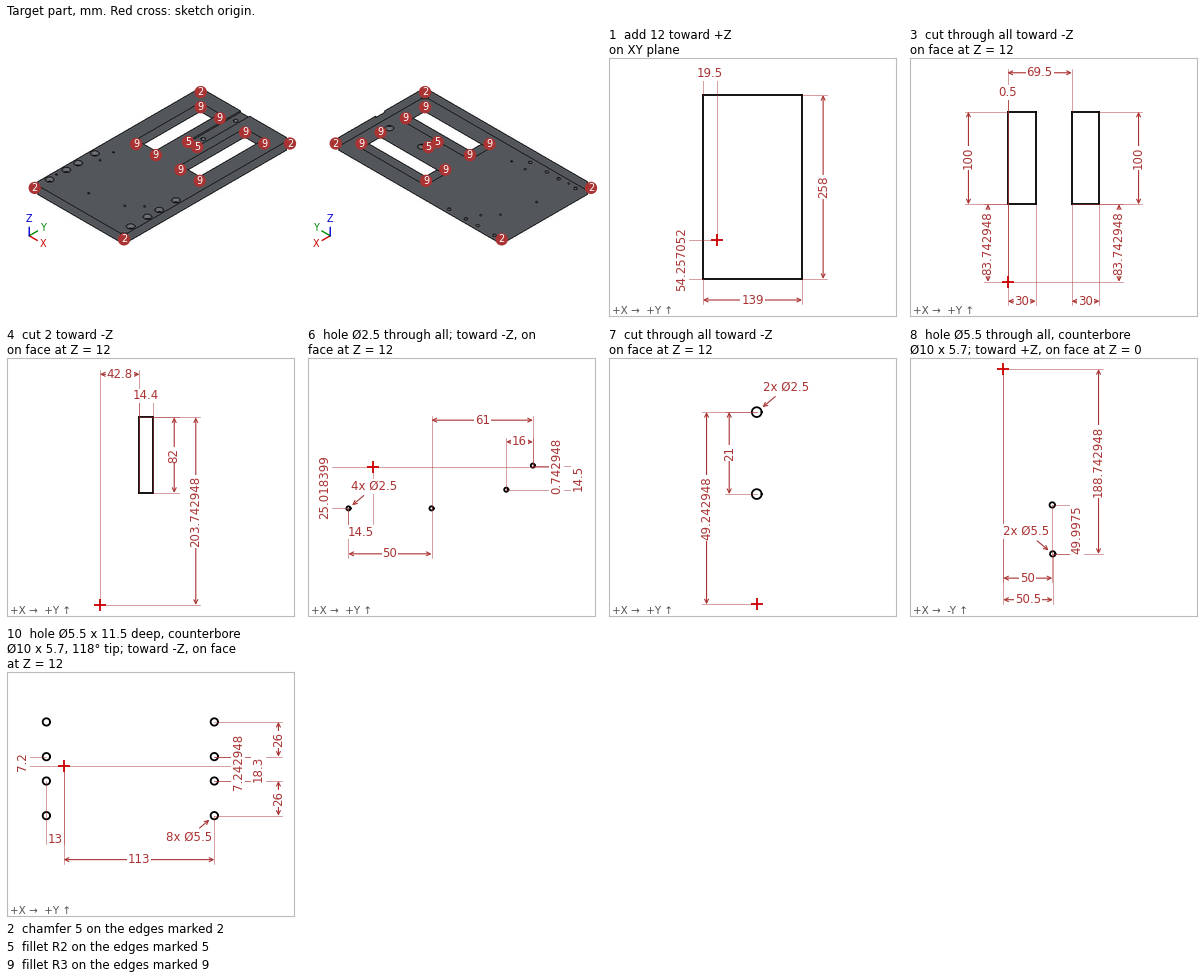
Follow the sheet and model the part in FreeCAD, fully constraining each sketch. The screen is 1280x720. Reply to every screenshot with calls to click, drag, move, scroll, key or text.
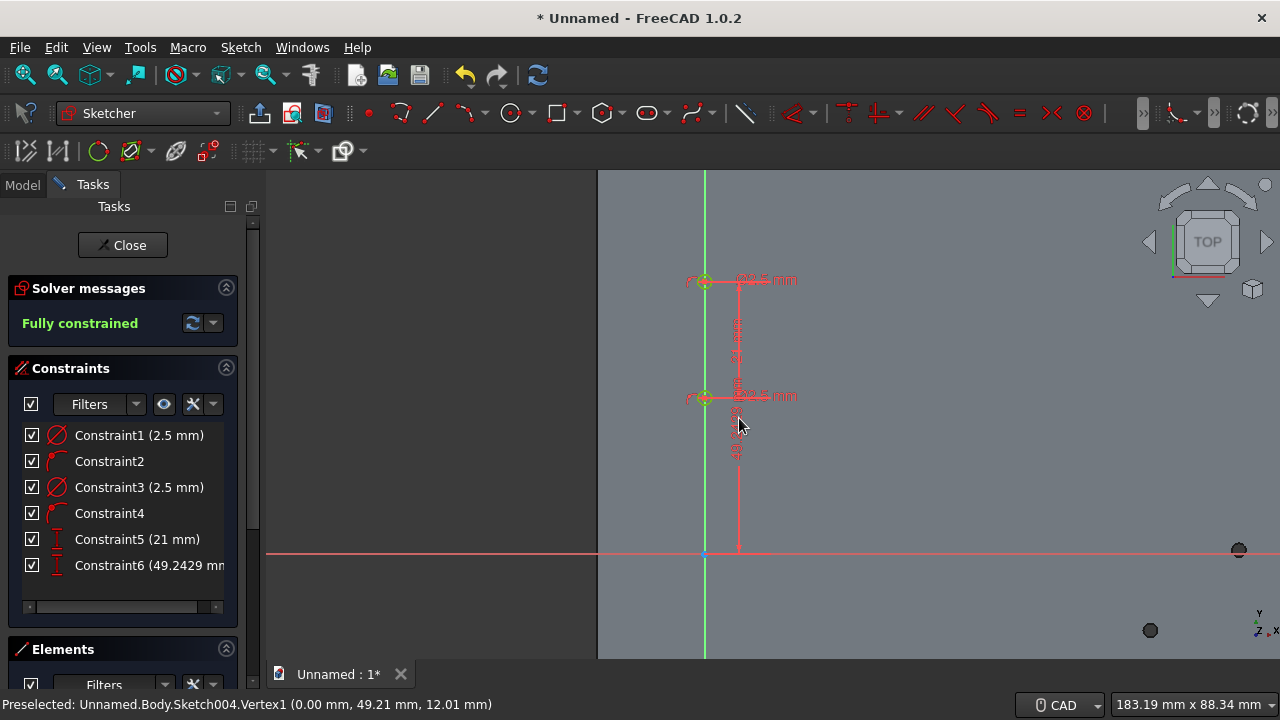
click(123, 245)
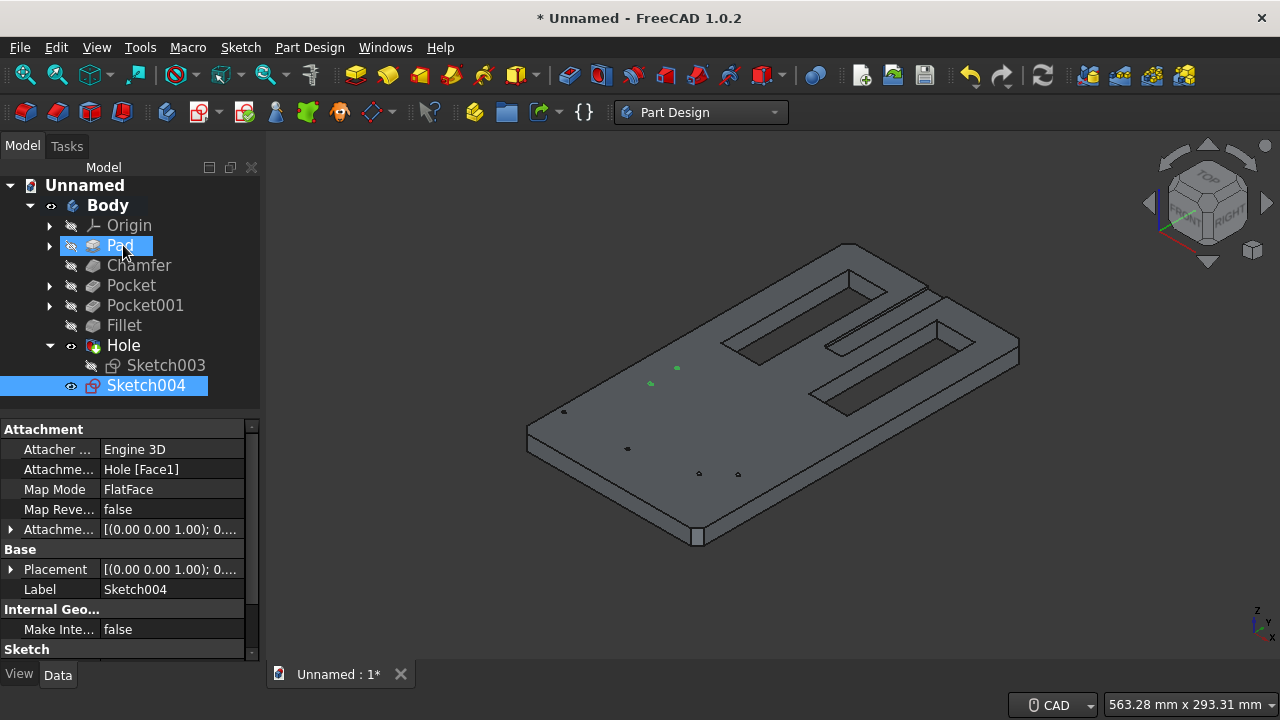
click(570, 76)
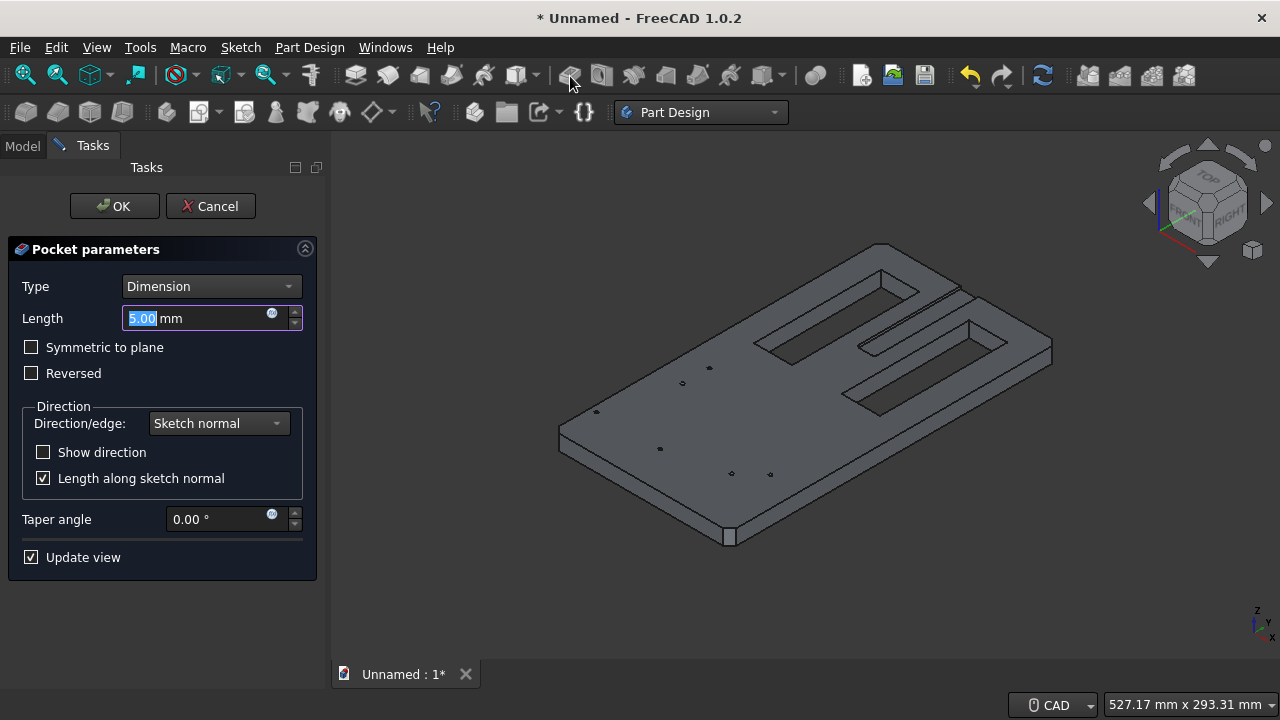
click(212, 286)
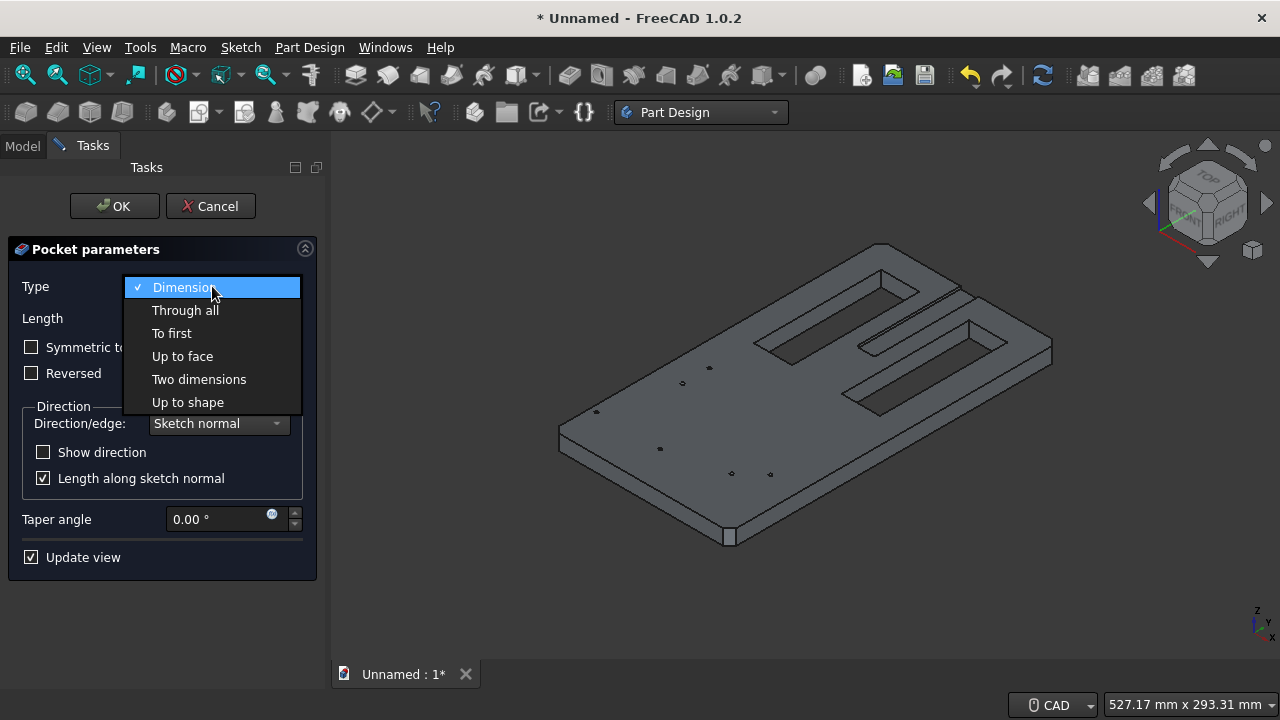
click(212, 310)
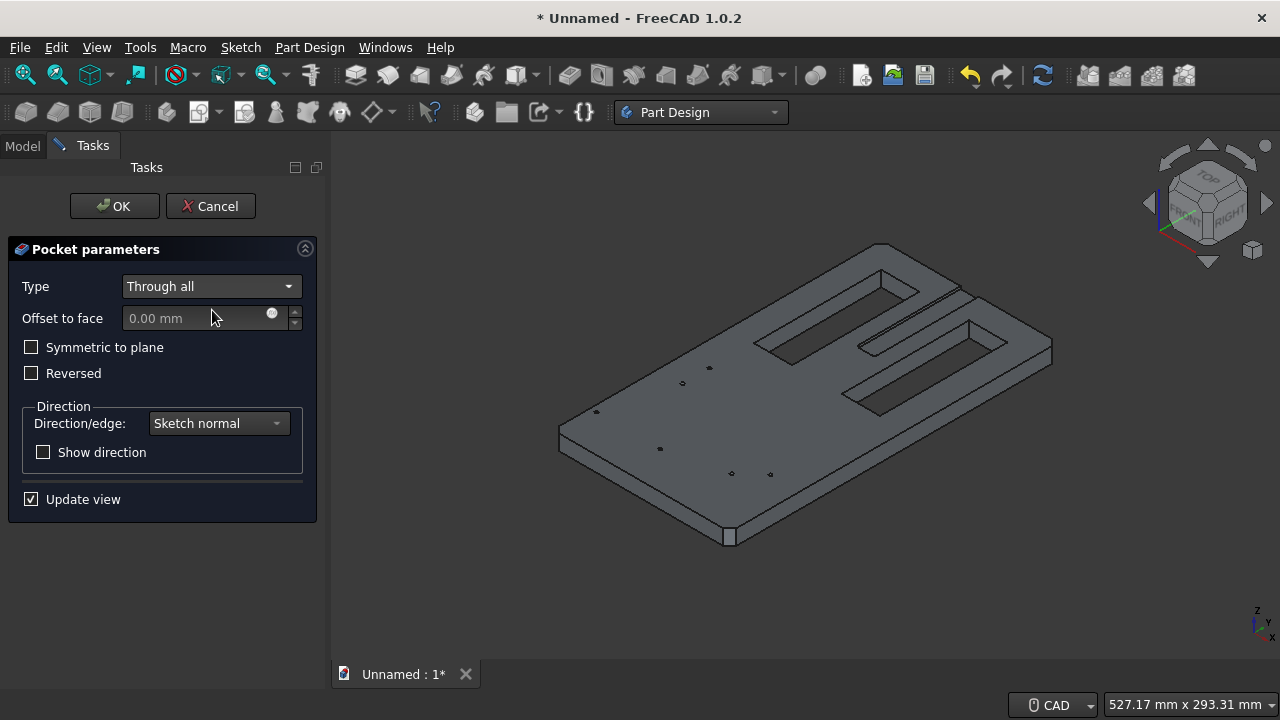
click(115, 206)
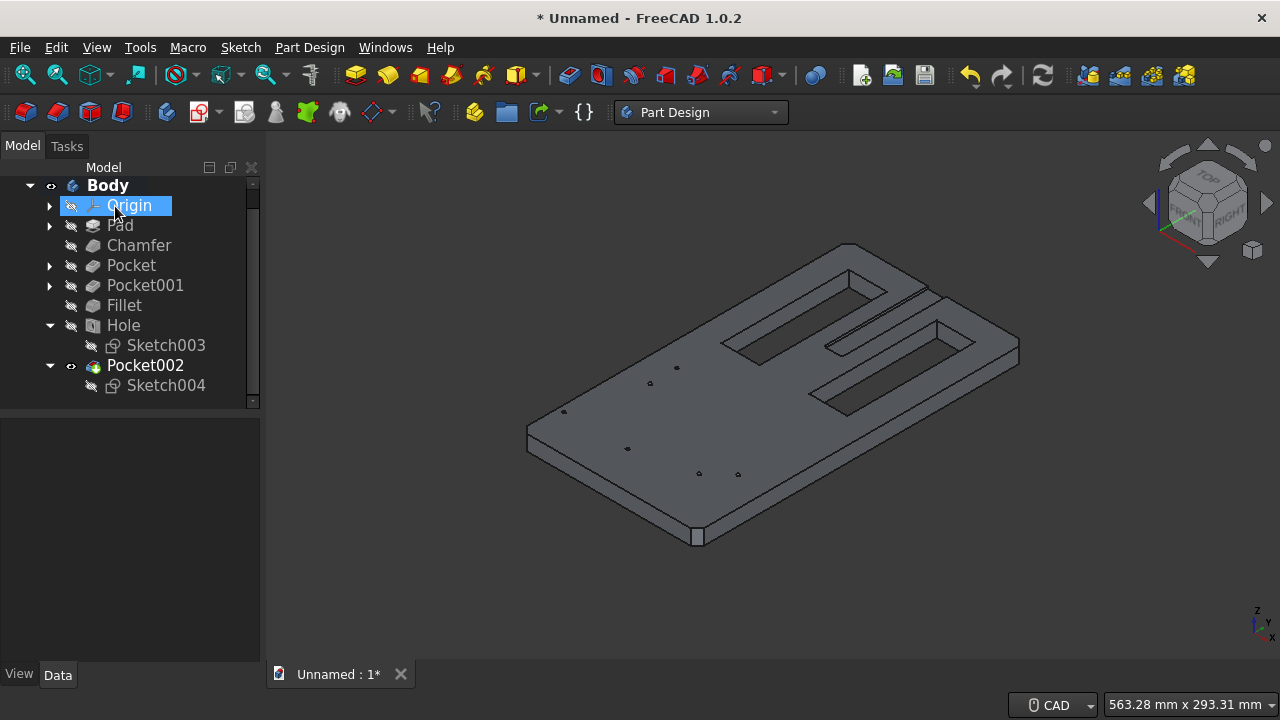
key(5)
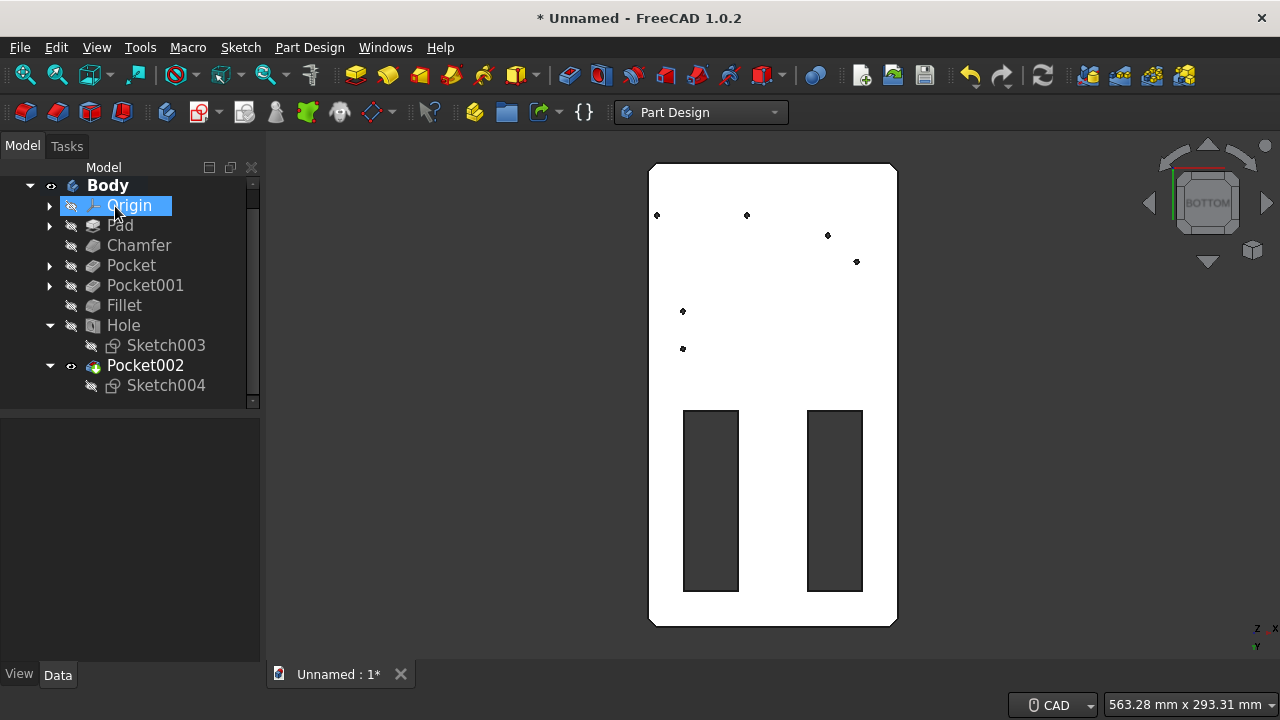
click(773, 328)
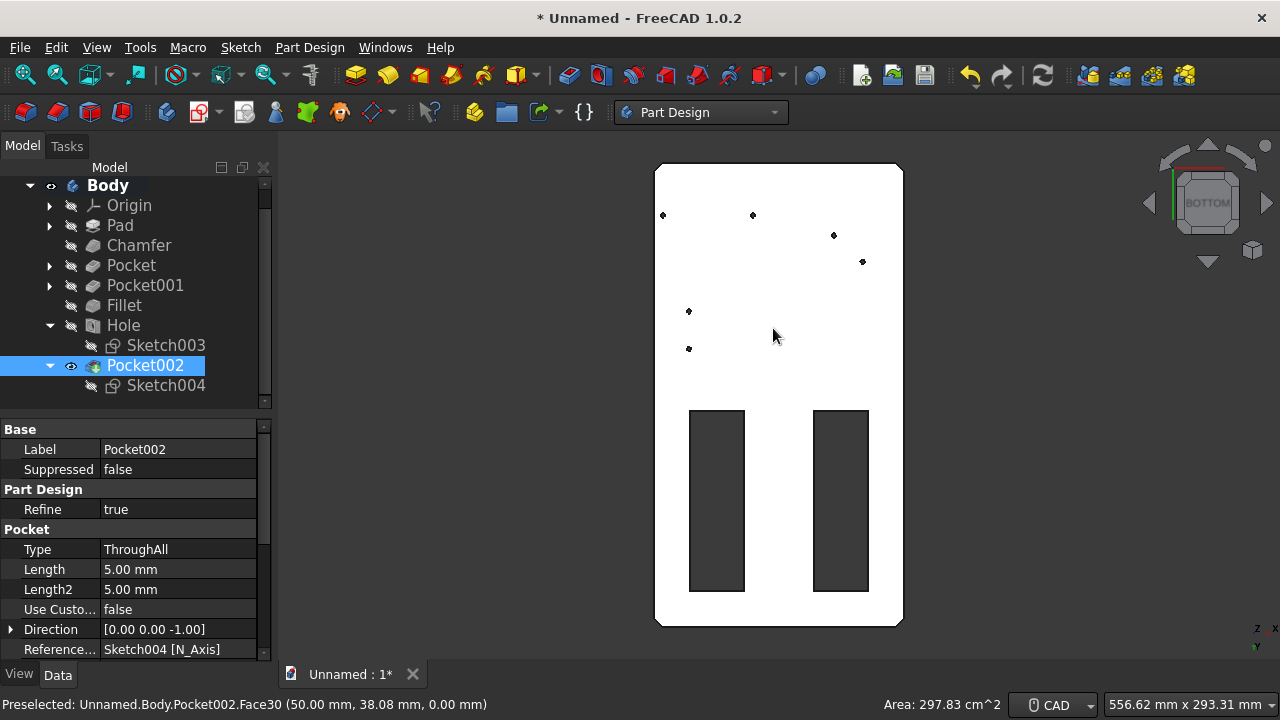
click(200, 112)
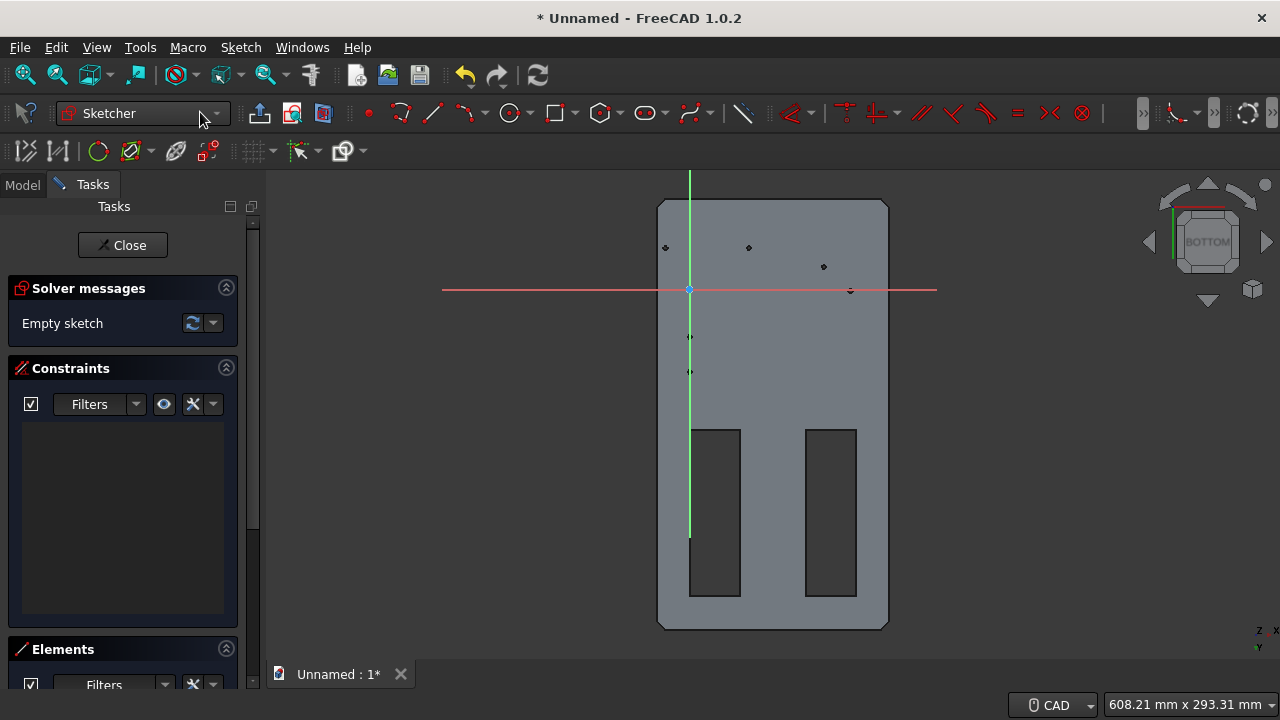
scroll(803, 627, up, 6)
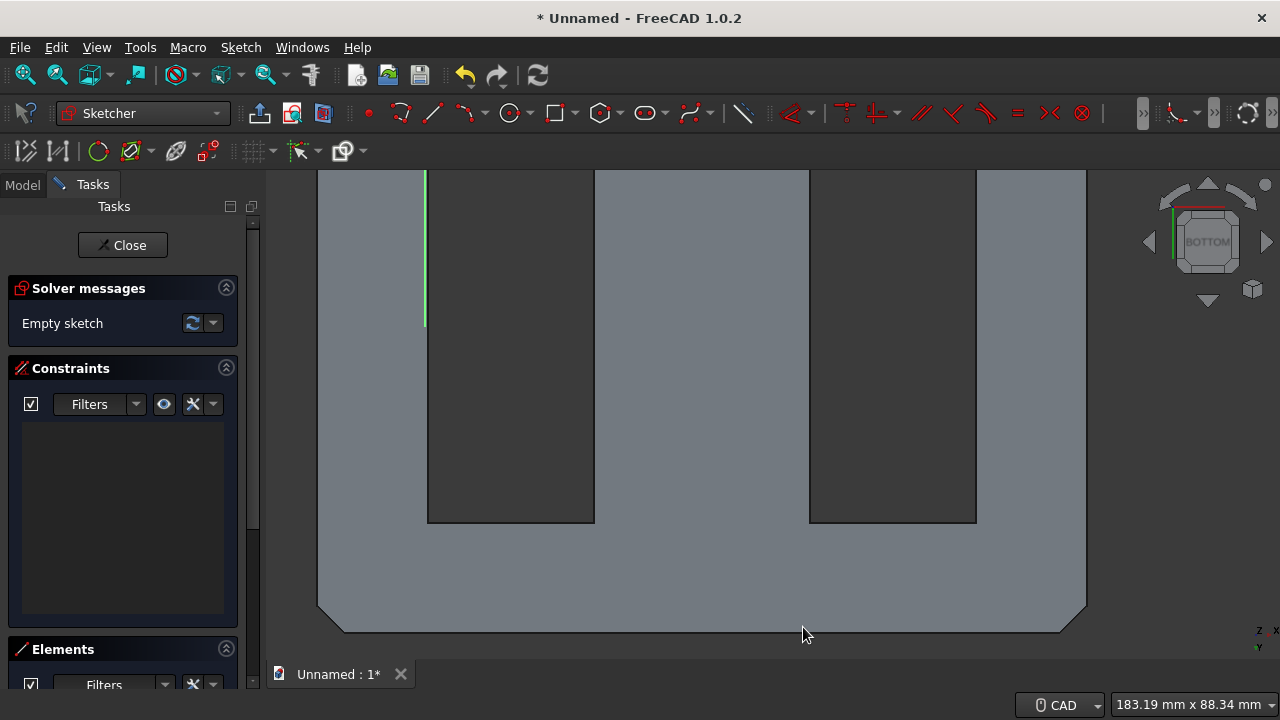
key(g)
key(c)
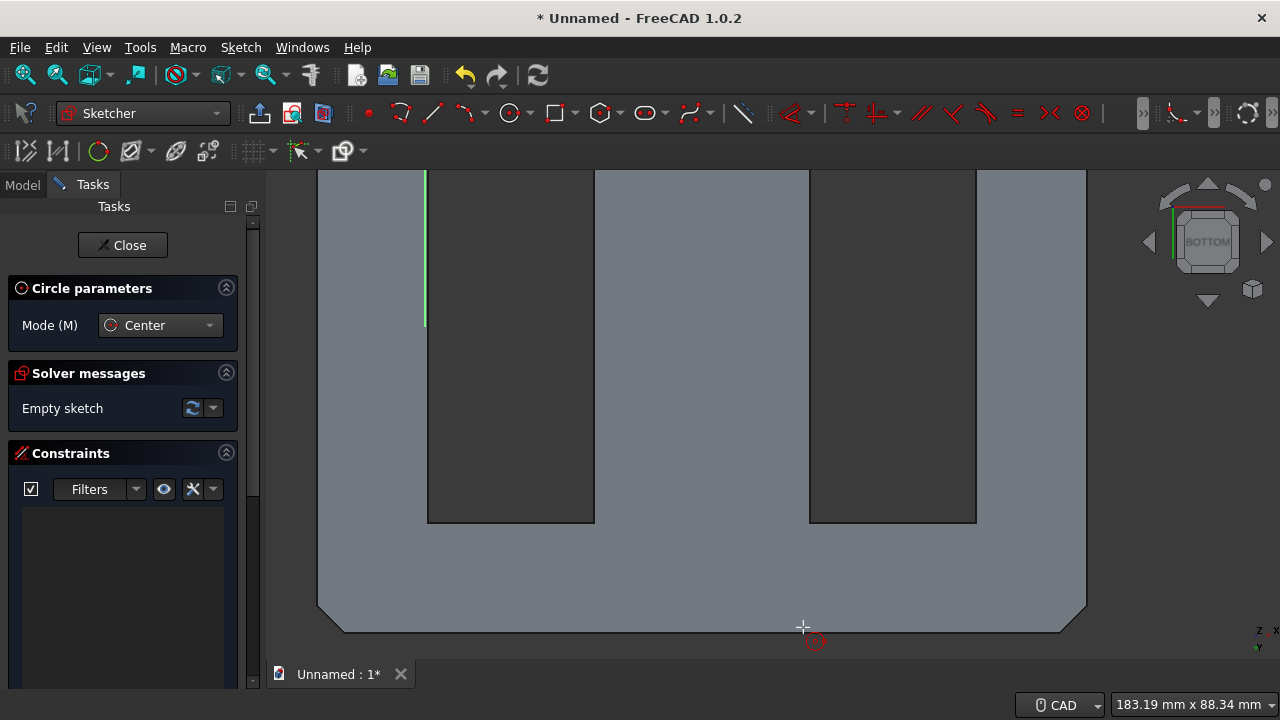
scroll(705, 550, up, 2)